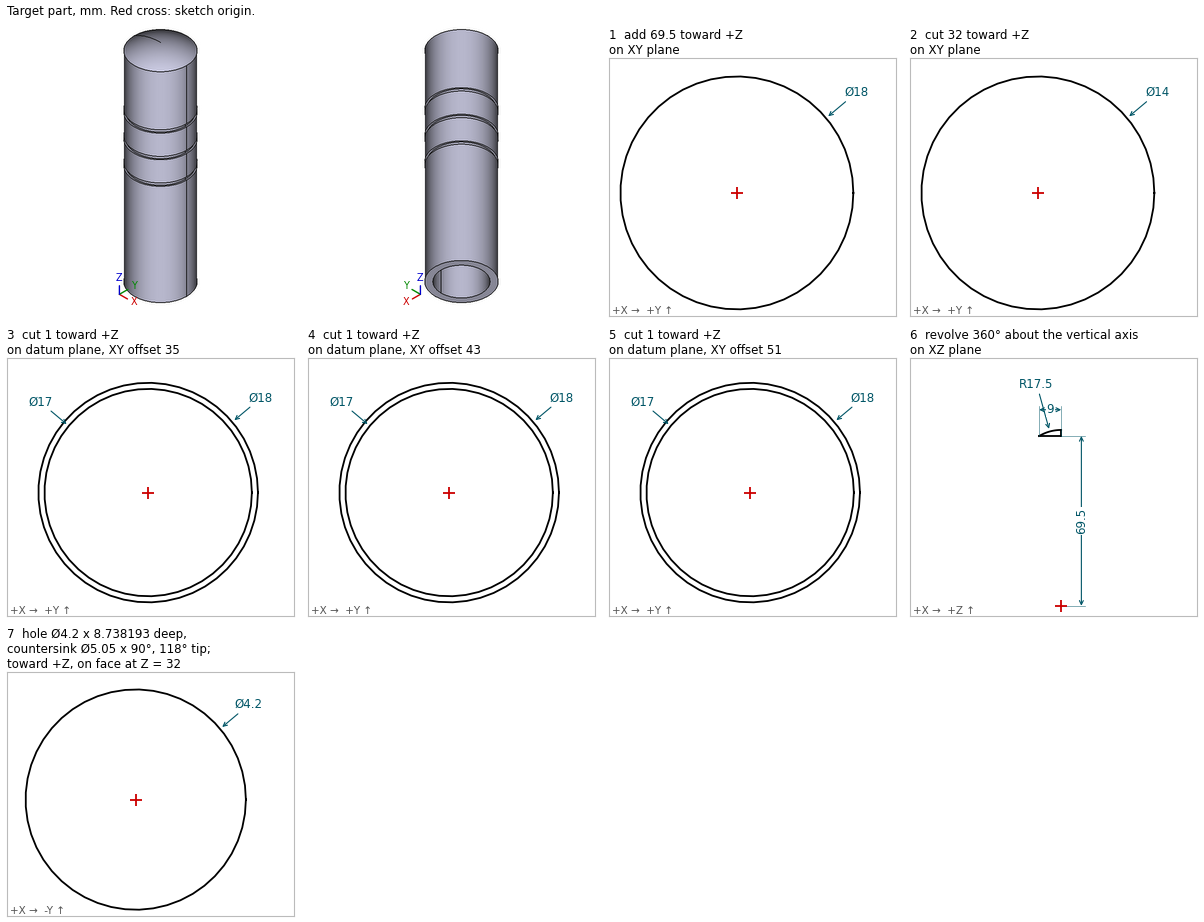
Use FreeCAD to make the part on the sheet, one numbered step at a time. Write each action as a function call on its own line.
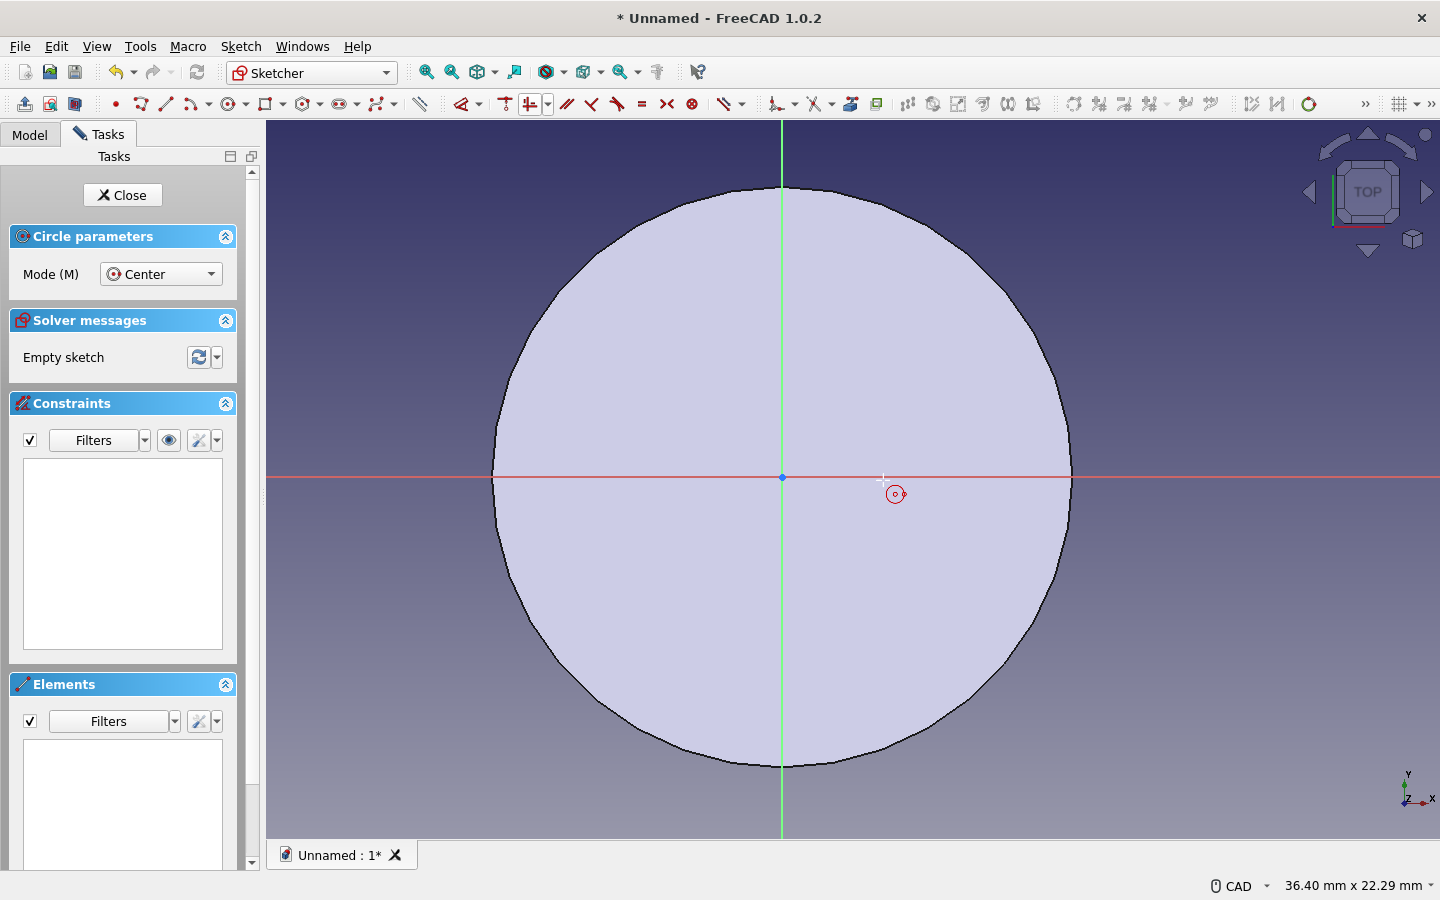
click(782, 477)
click(942, 318)
key(Escape)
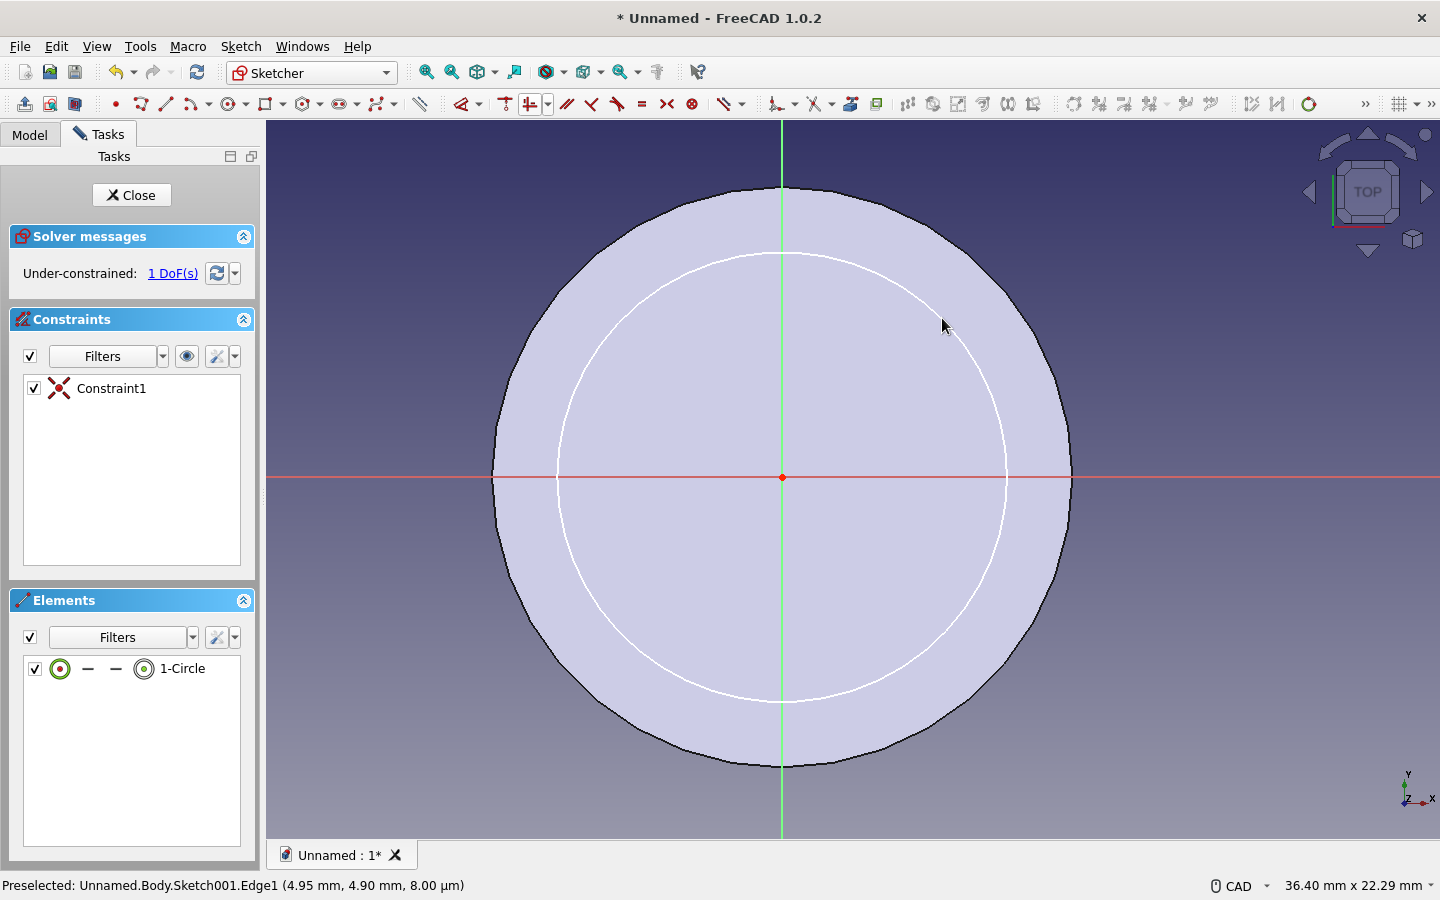
key(d)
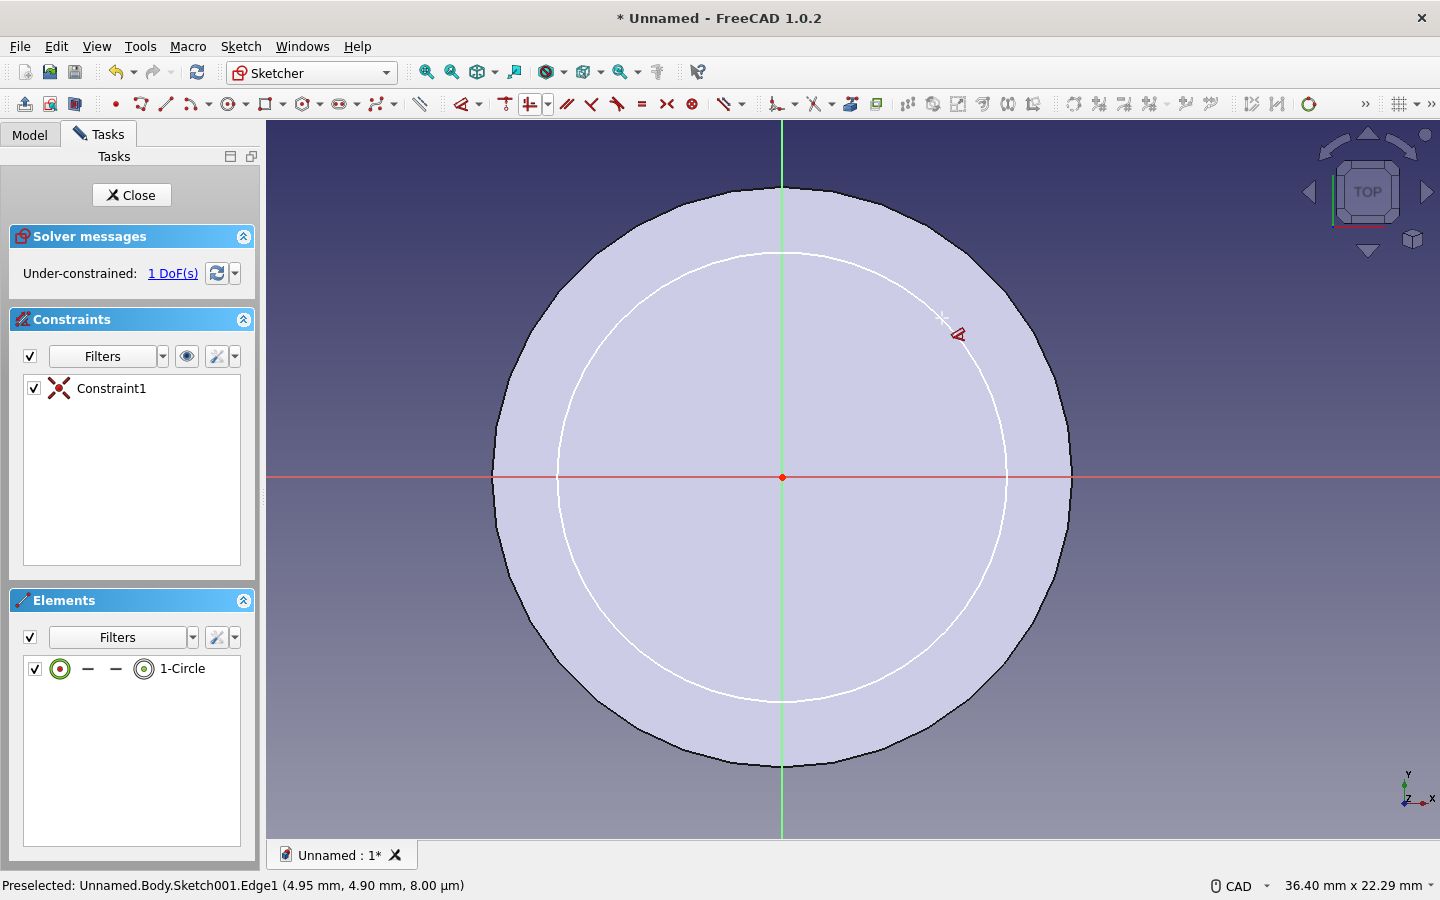
click(941, 318)
click(964, 295)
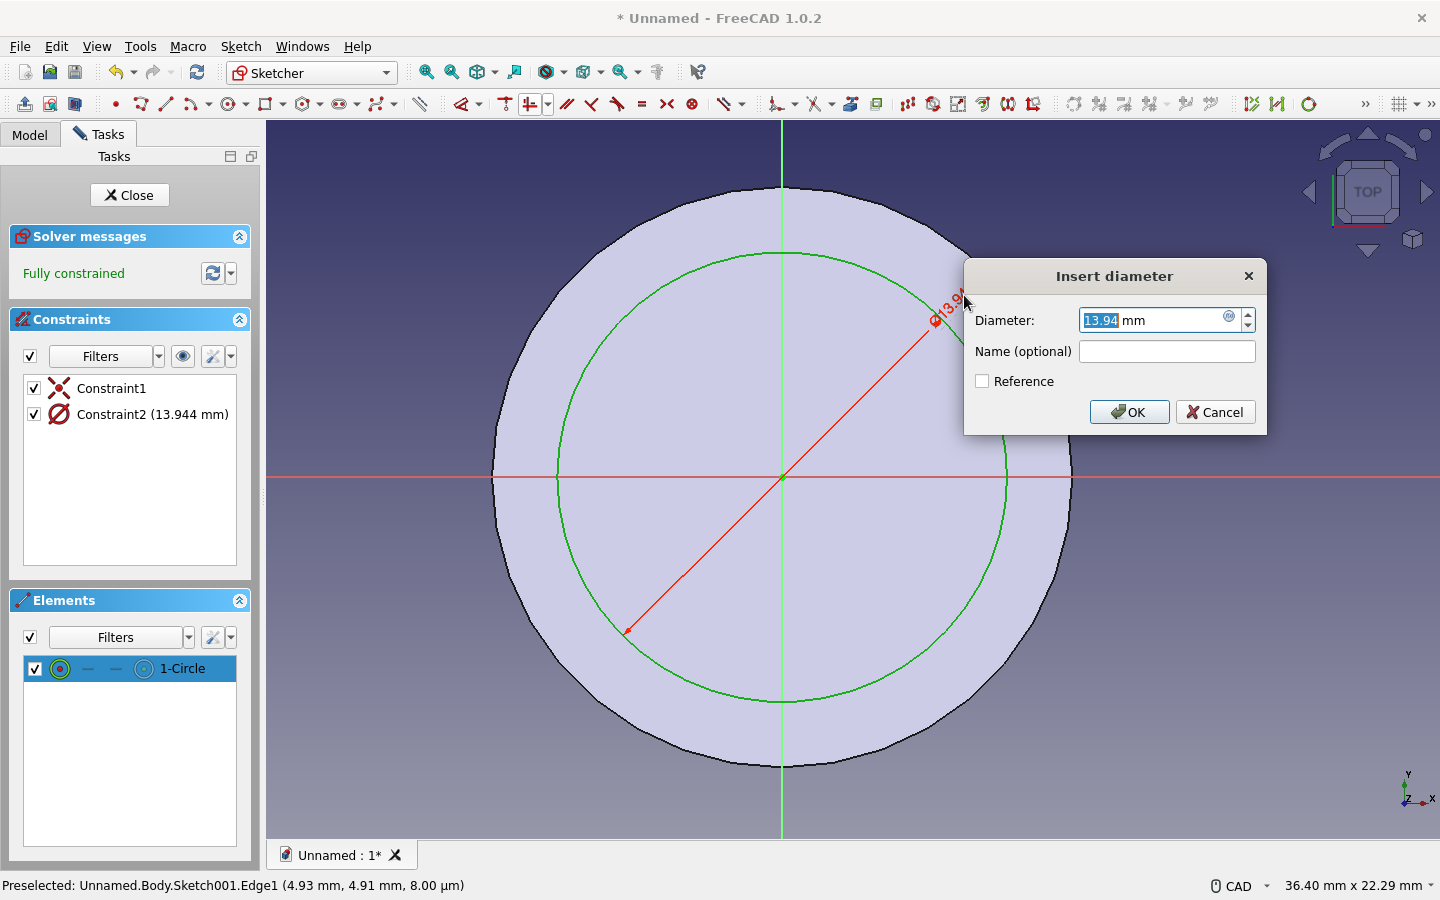
text(14)
key(Return)
key(Escape)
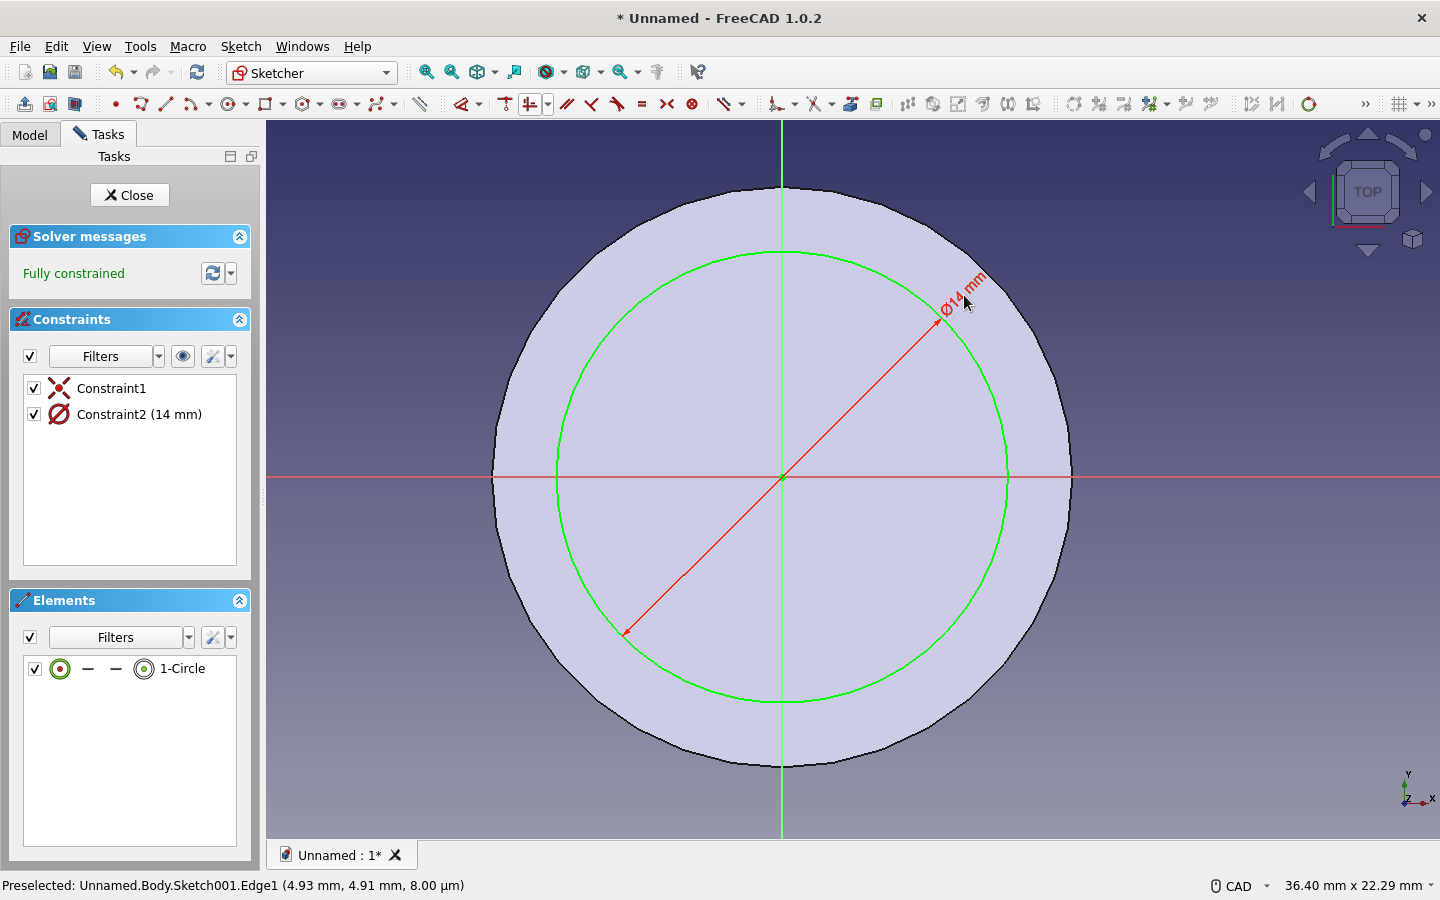
click(130, 195)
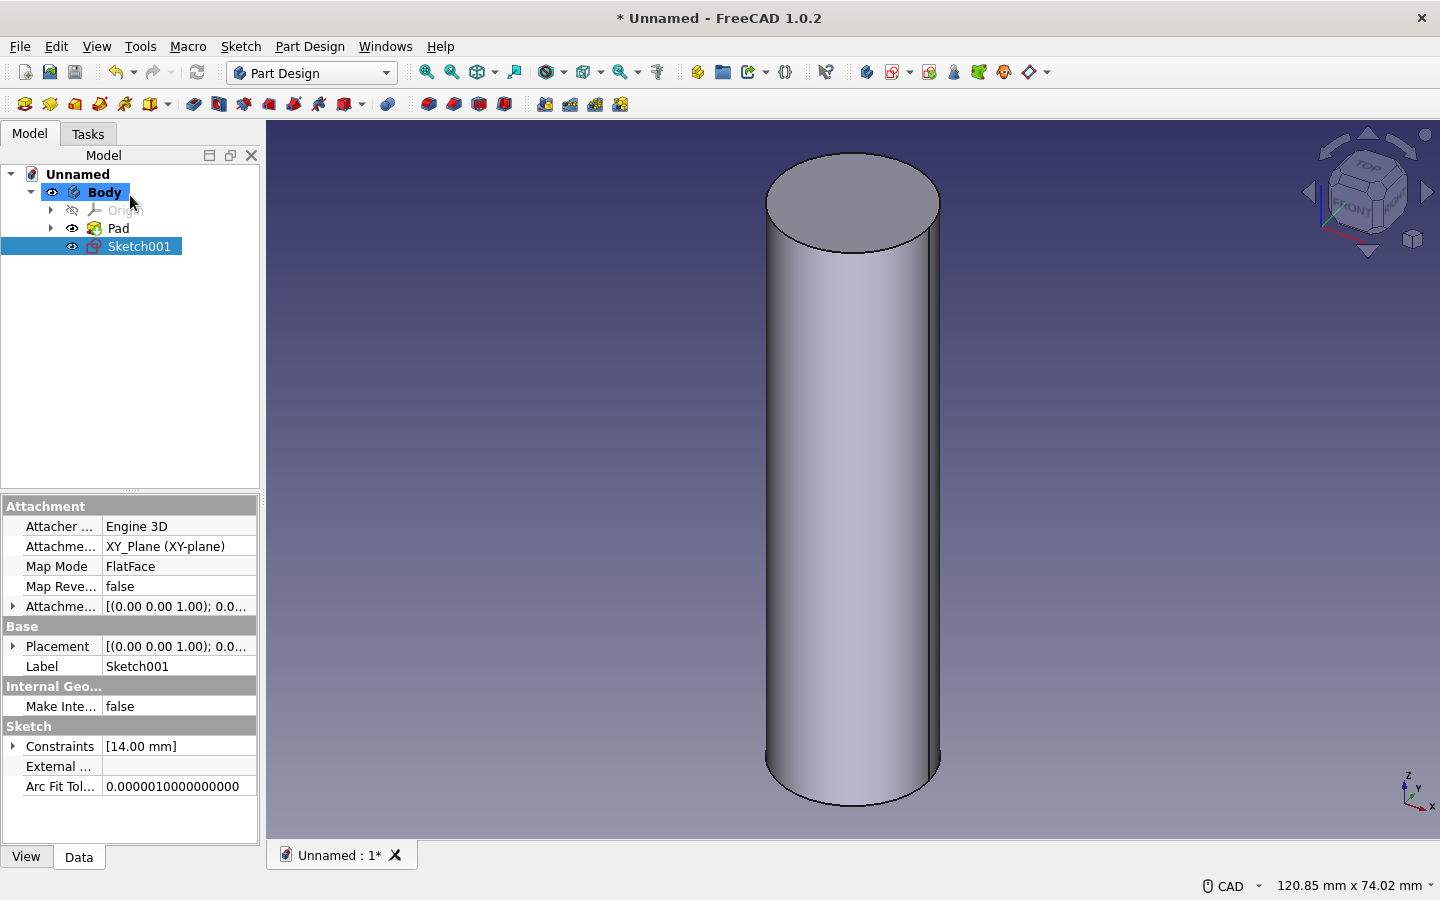
click(194, 104)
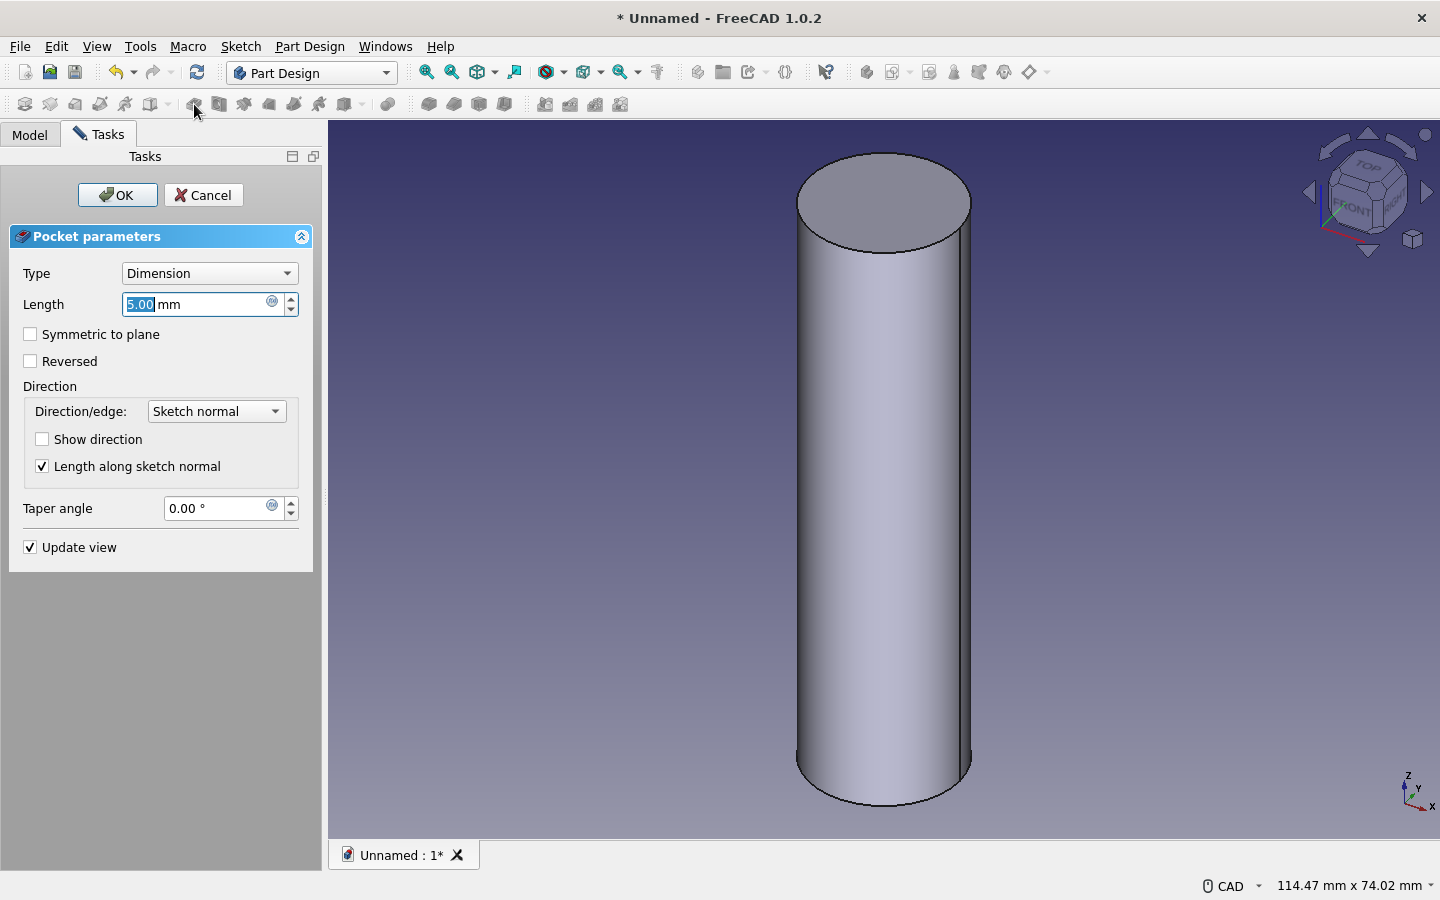
text(32)
key(Tab)